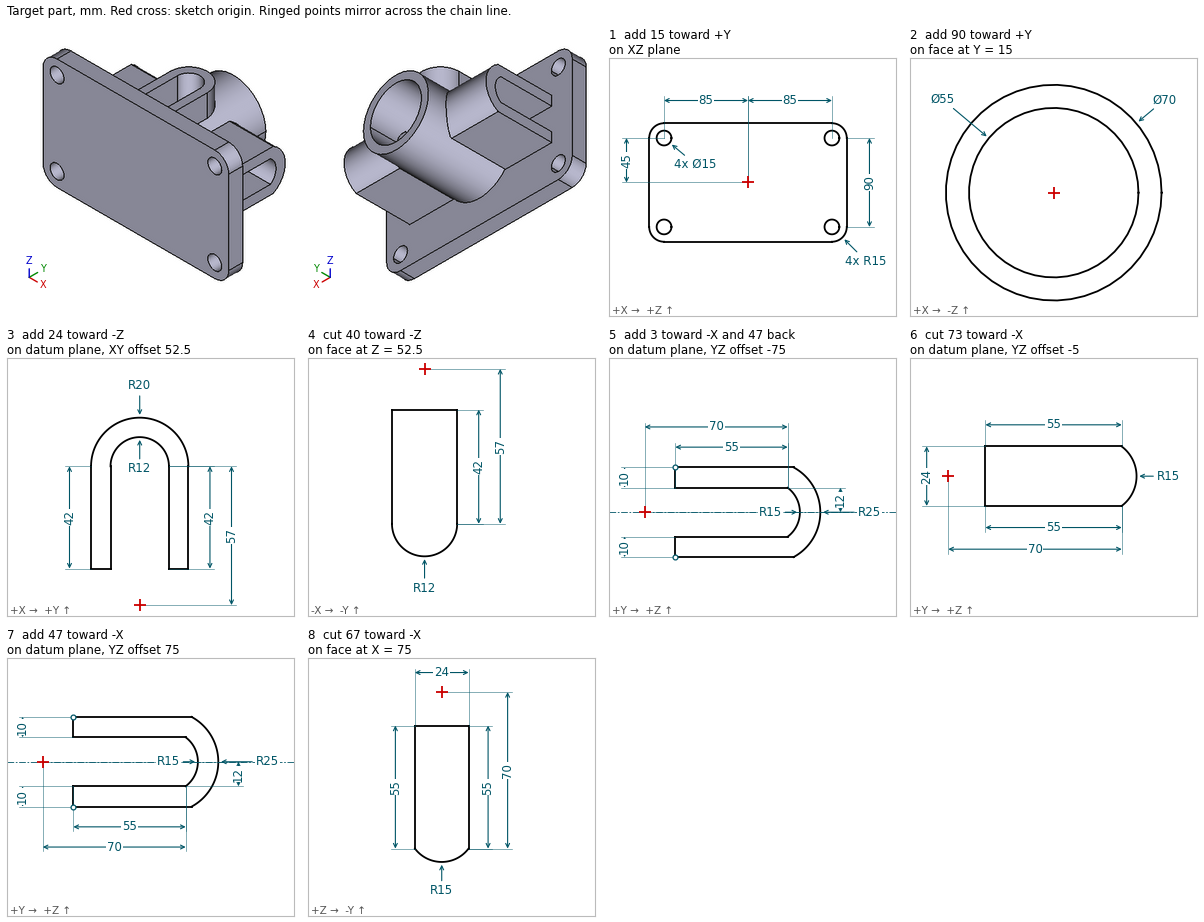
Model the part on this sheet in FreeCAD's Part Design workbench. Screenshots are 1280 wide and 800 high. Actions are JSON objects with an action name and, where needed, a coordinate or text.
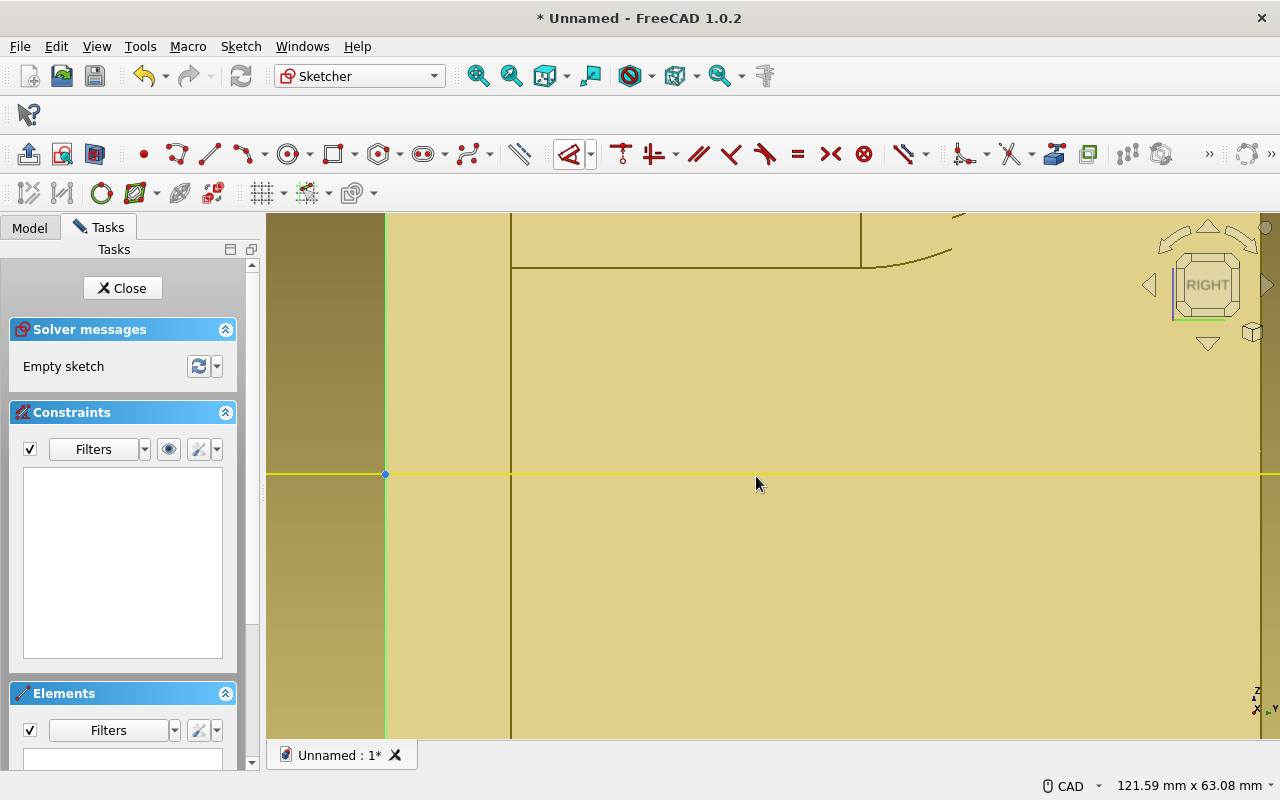
{"action": "key", "text": "g m"}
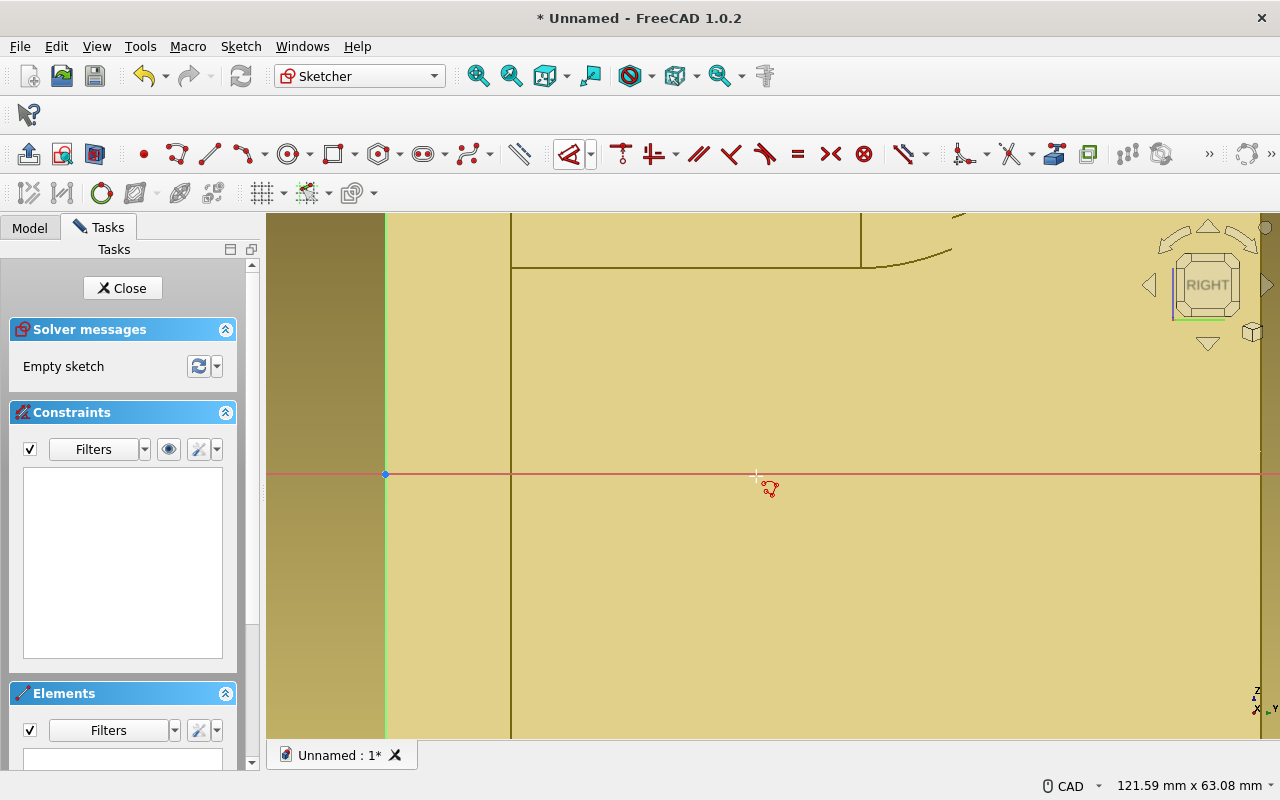
{"action": "left_click", "coordinate": [969, 575]}
{"action": "left_click", "coordinate": [511, 575]}
{"action": "left_click", "coordinate": [511, 374]}
{"action": "left_click", "coordinate": [969, 374]}
{"action": "right_click", "coordinate": [969, 374]}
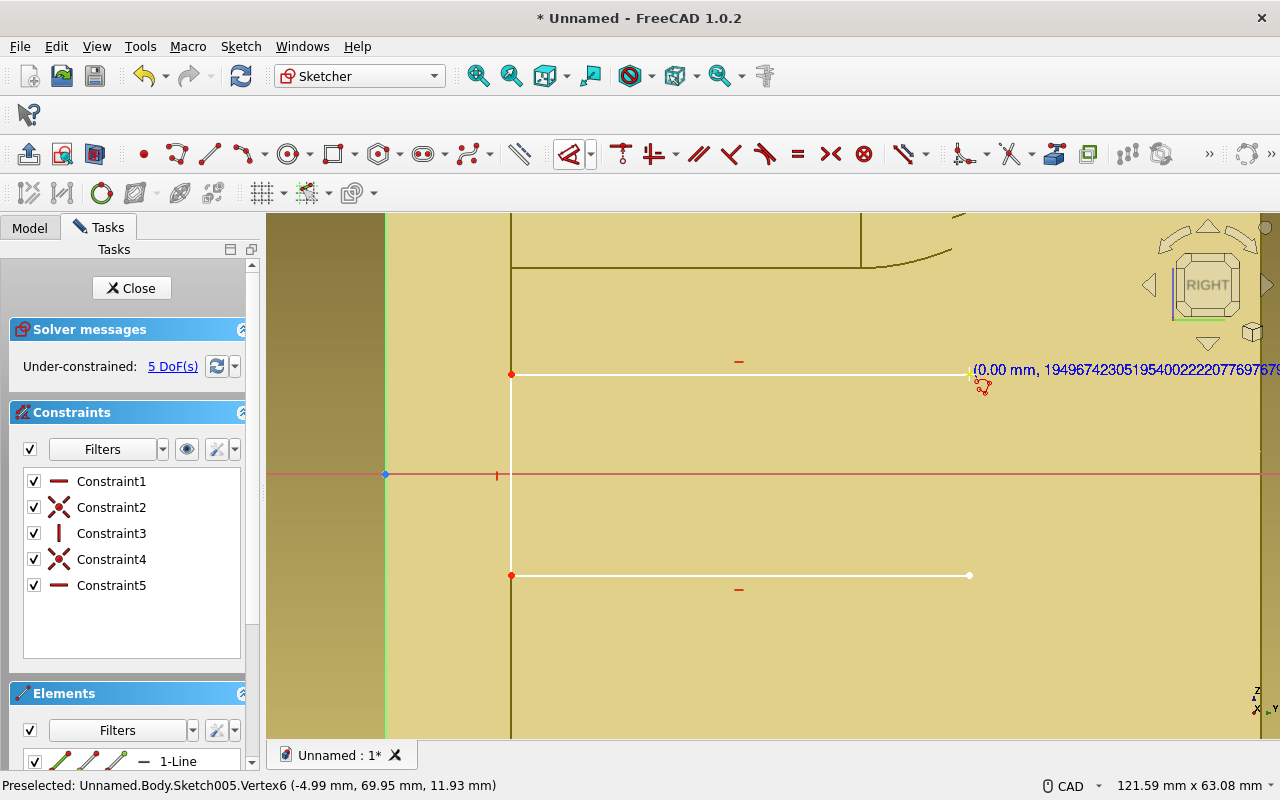
{"action": "key", "text": "g 3 a"}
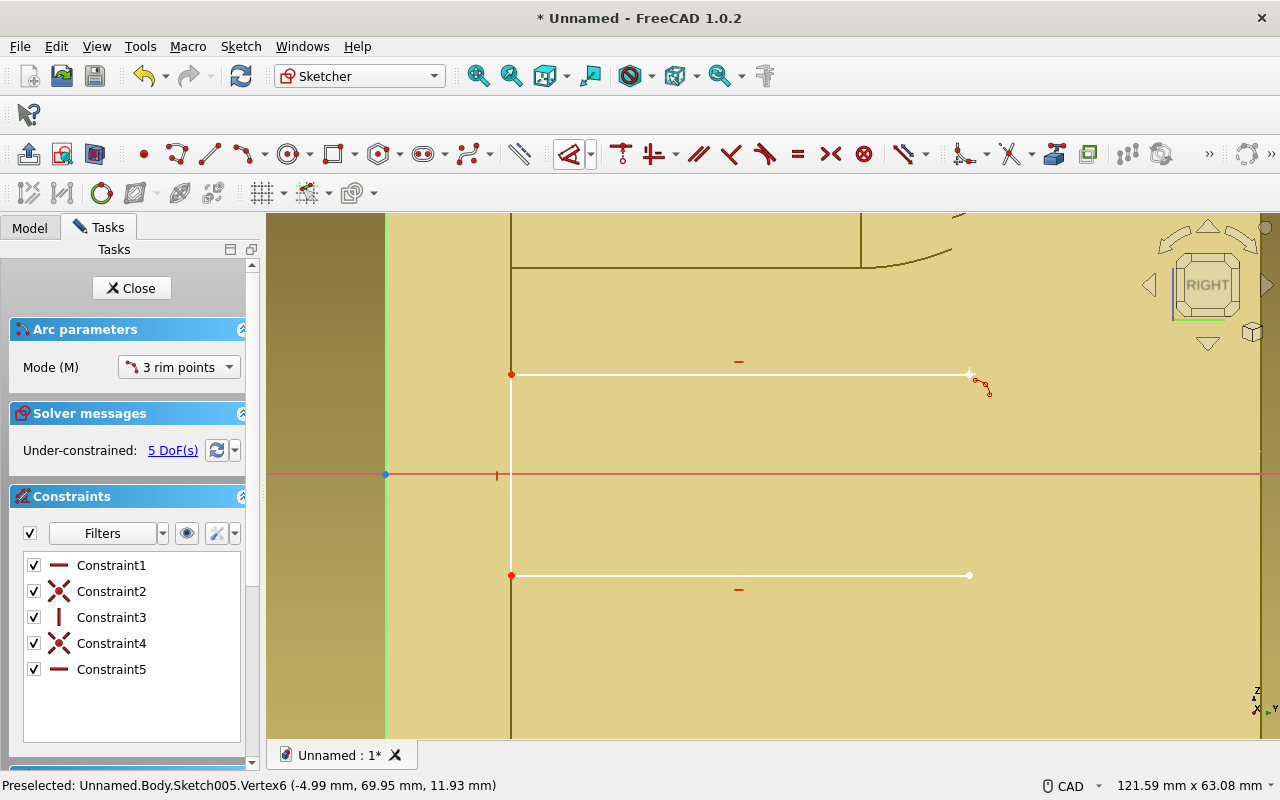
{"action": "left_click", "coordinate": [969, 375]}
{"action": "left_click", "coordinate": [969, 576]}
{"action": "left_click", "coordinate": [1017, 498]}
{"action": "key", "text": "Escape"}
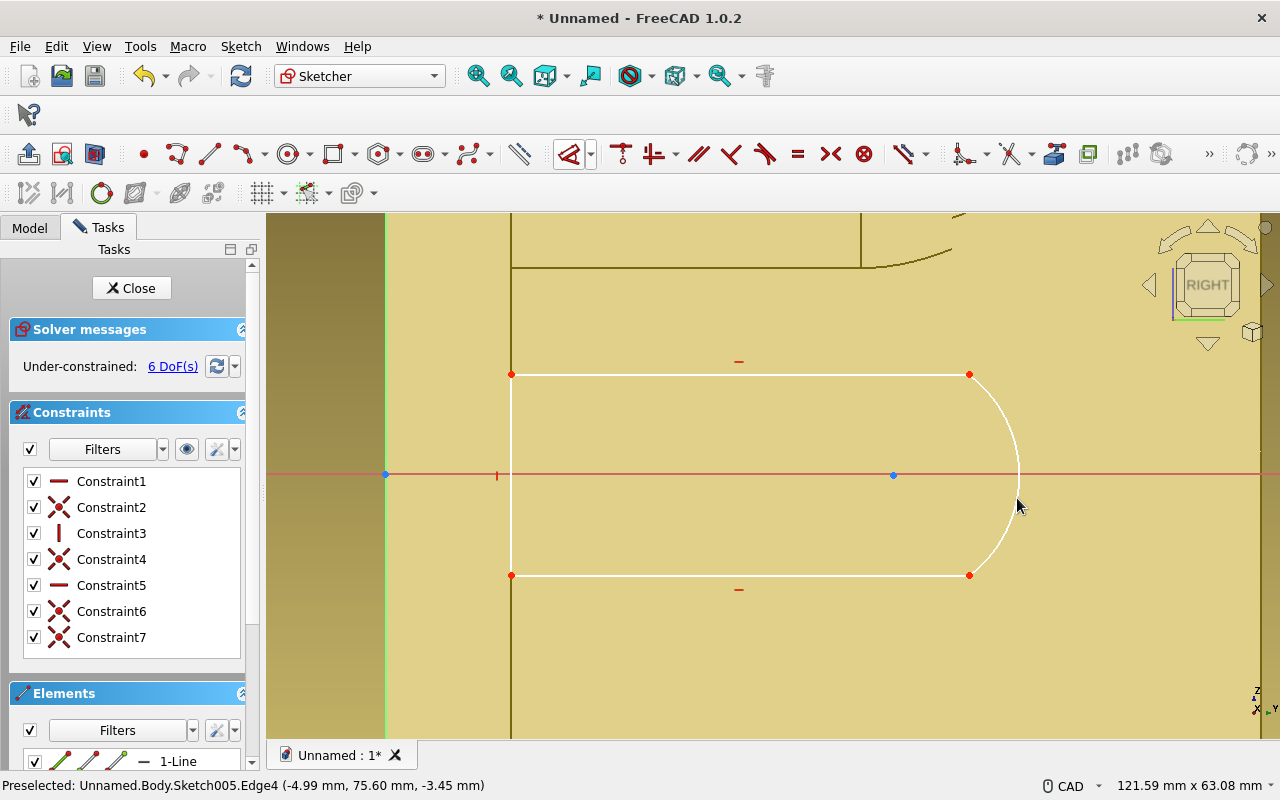
{"action": "left_click", "coordinate": [894, 475]}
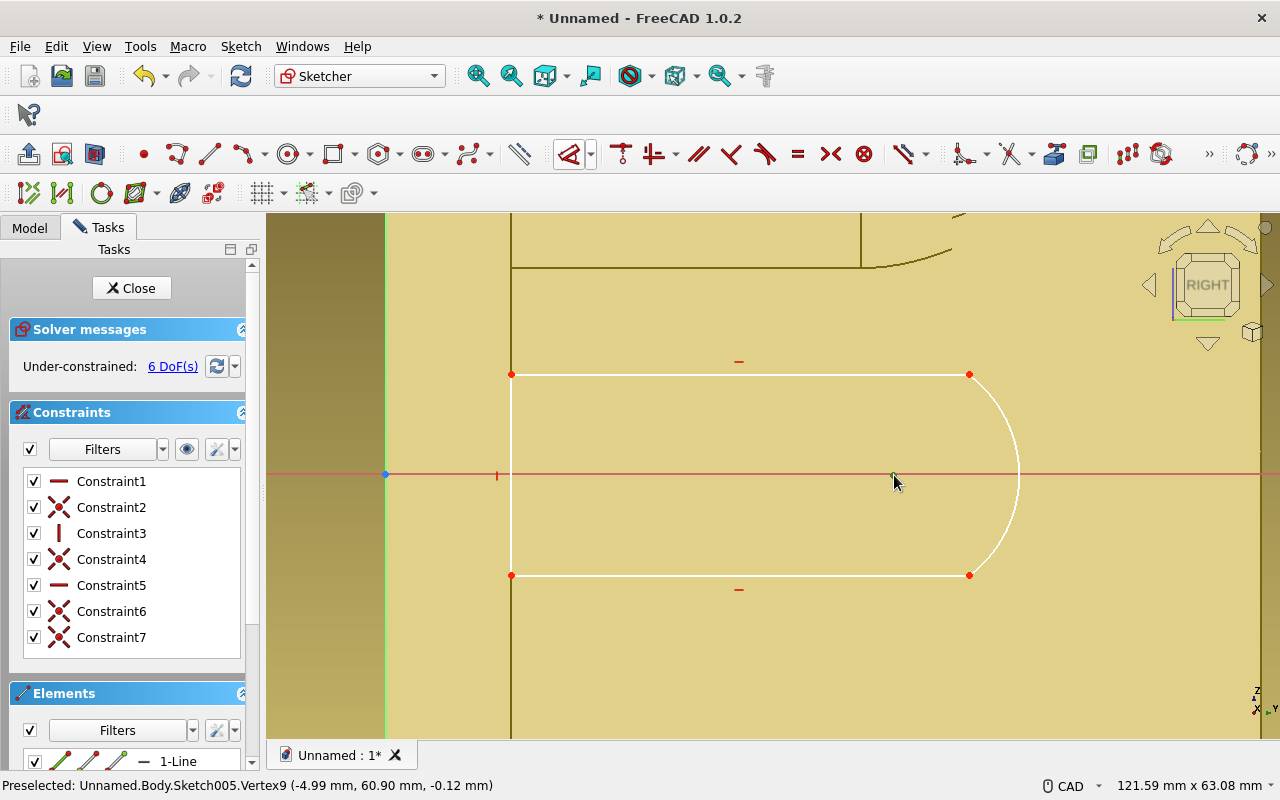
{"action": "left_click", "coordinate": [353, 474]}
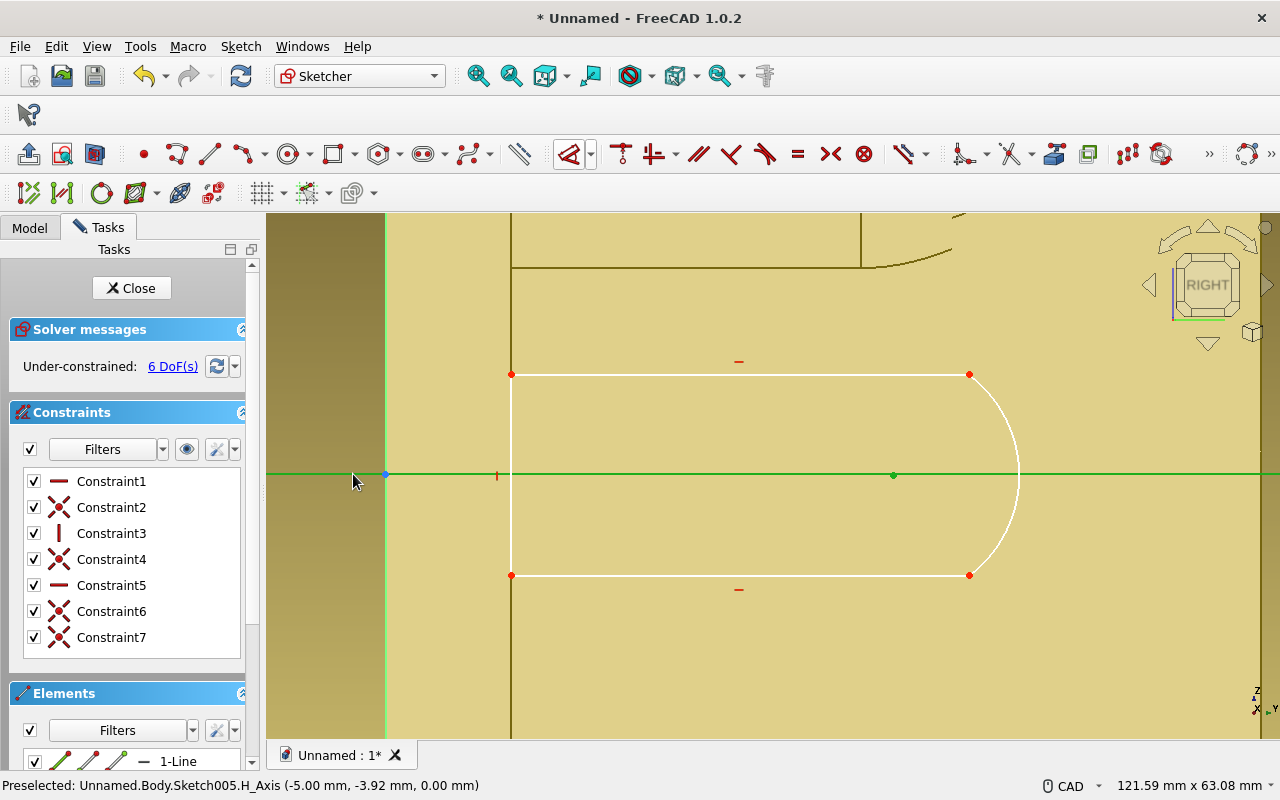
{"action": "left_click", "coordinate": [621, 154]}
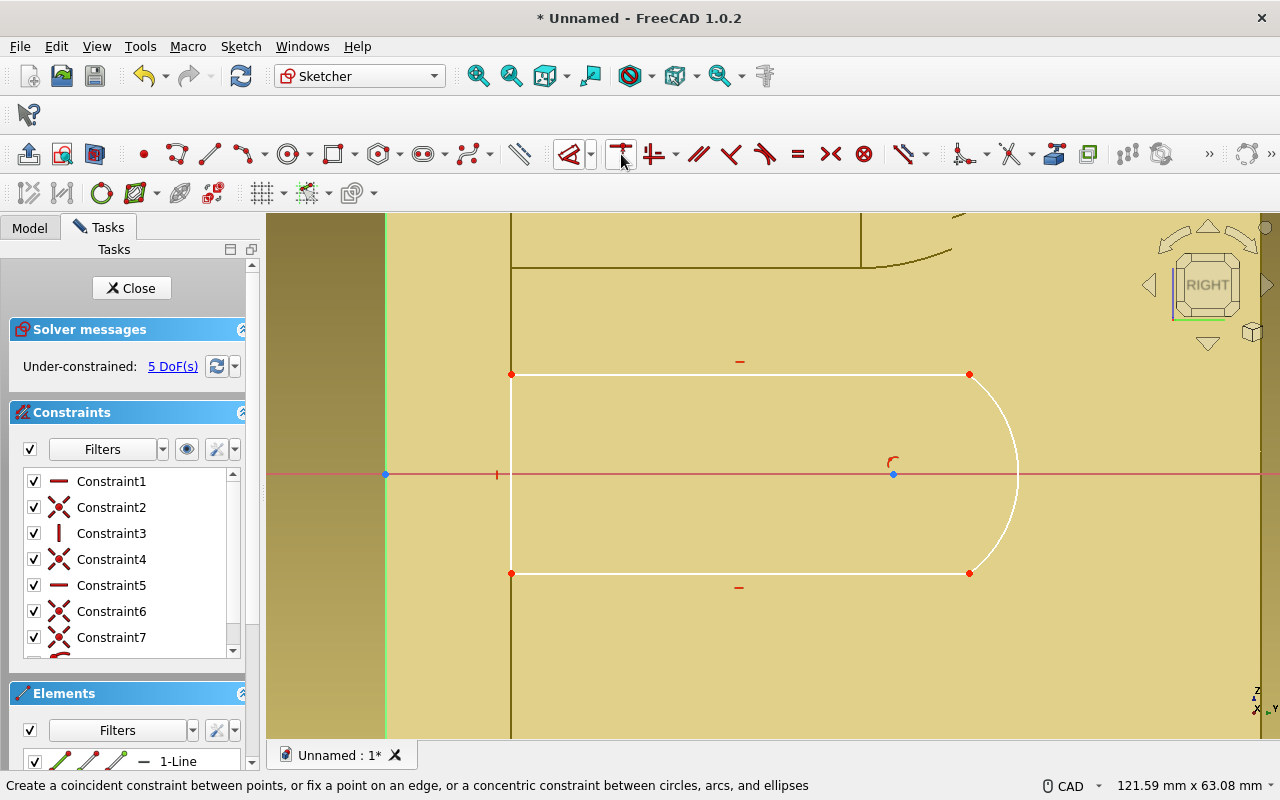
{"action": "left_click", "coordinate": [1010, 519]}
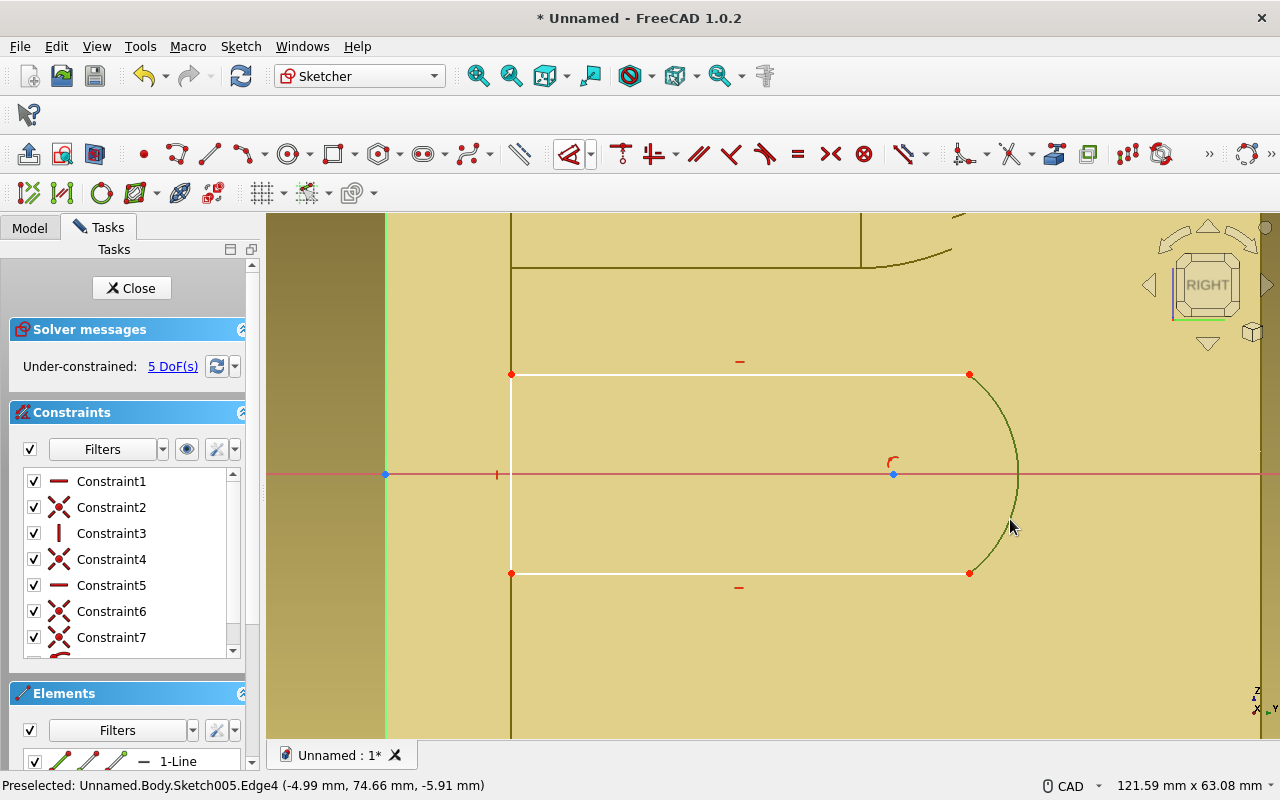
{"action": "key", "text": "k r"}